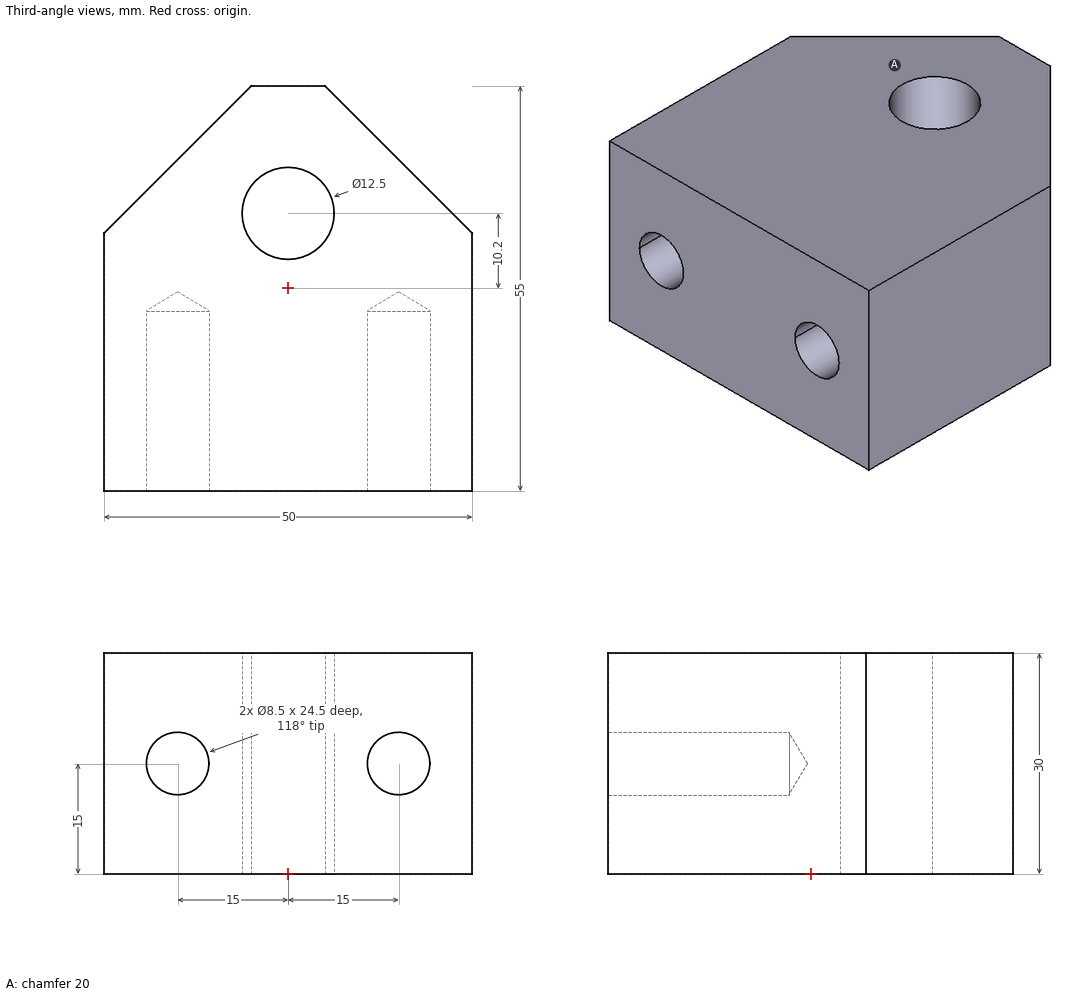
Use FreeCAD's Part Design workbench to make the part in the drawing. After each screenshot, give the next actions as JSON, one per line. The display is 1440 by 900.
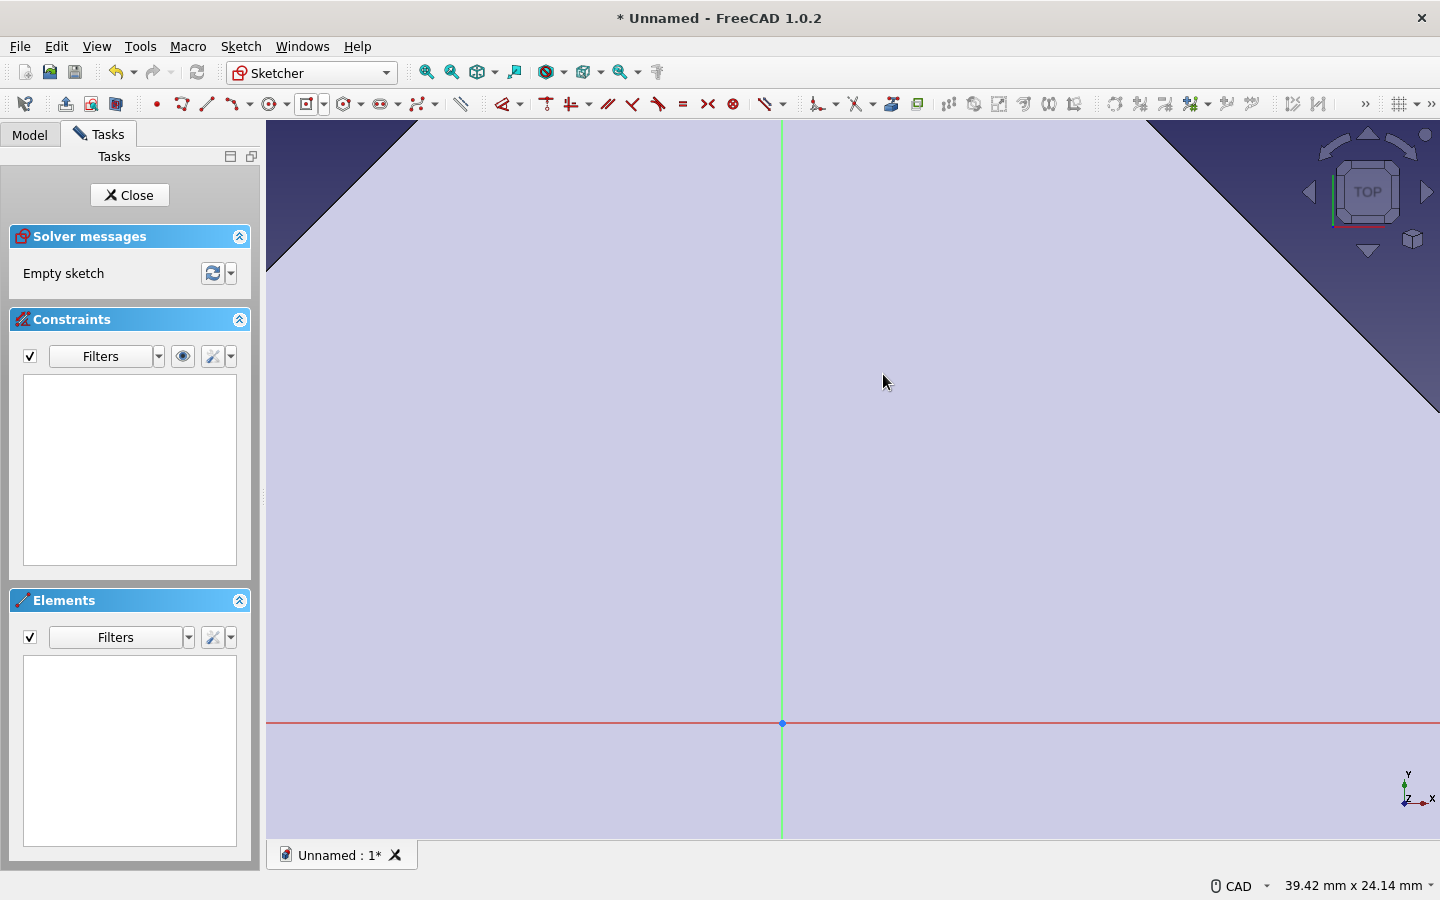
{"action": "left_click", "coordinate": [268, 104]}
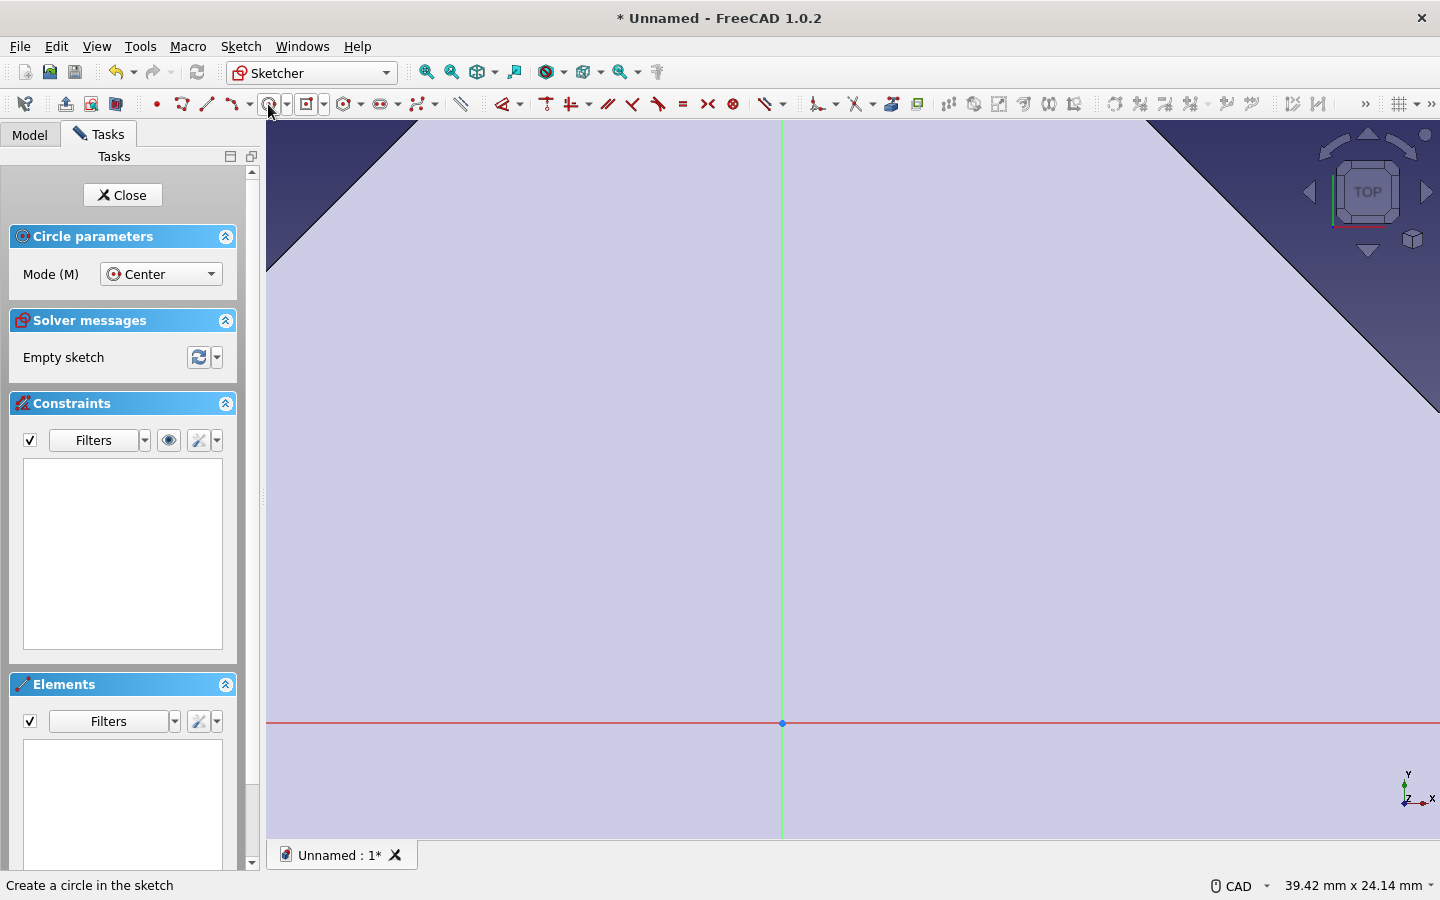
{"action": "left_click", "coordinate": [782, 420]}
{"action": "mouse_move", "coordinate": [914, 288]}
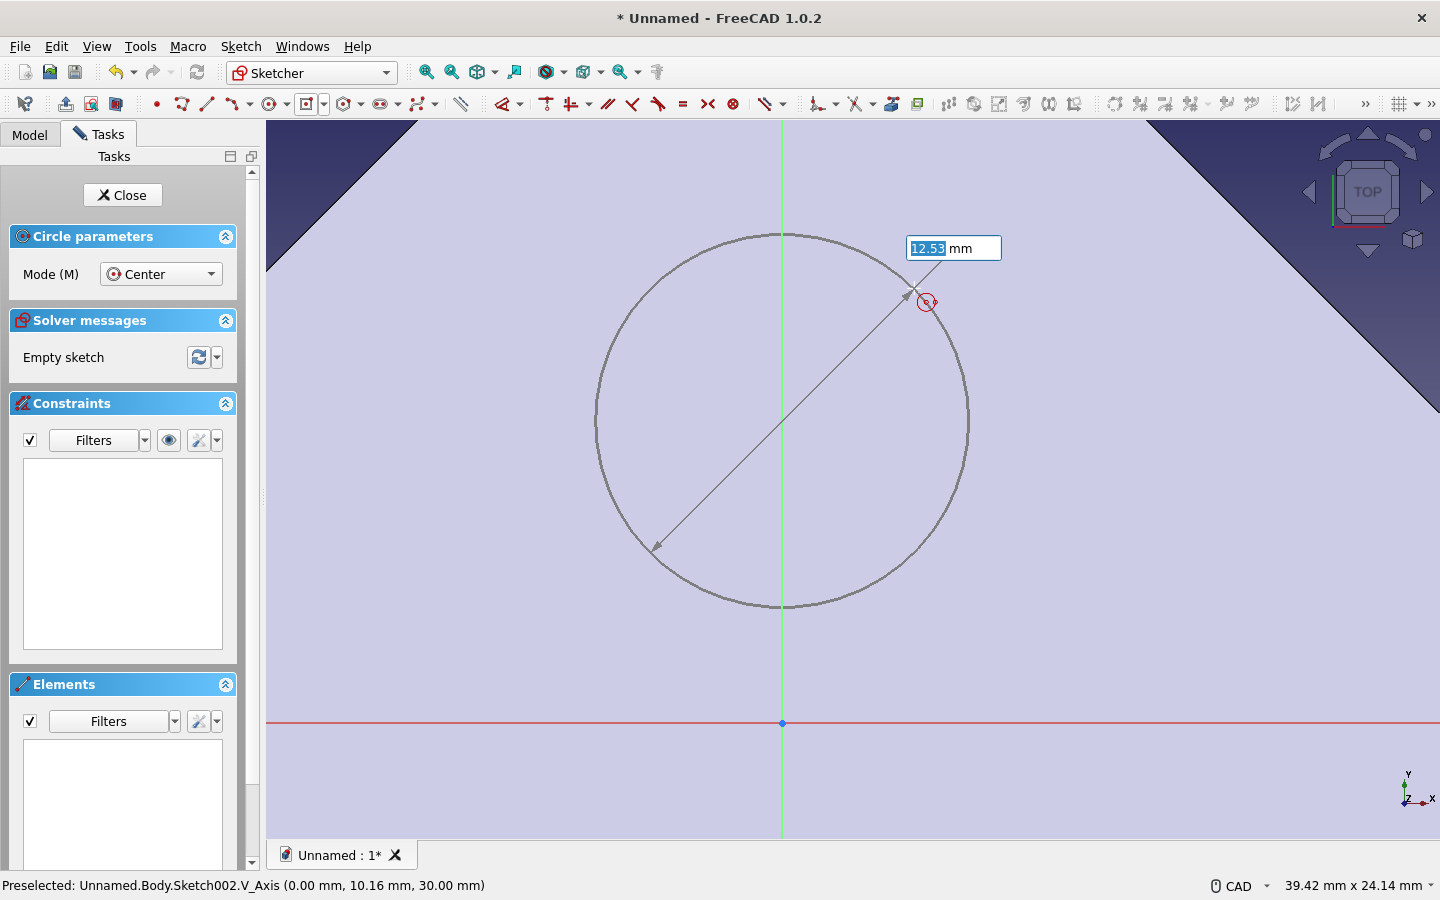
{"action": "type", "text": "12.5"}
{"action": "key", "text": "Return"}
{"action": "key", "text": "Escape"}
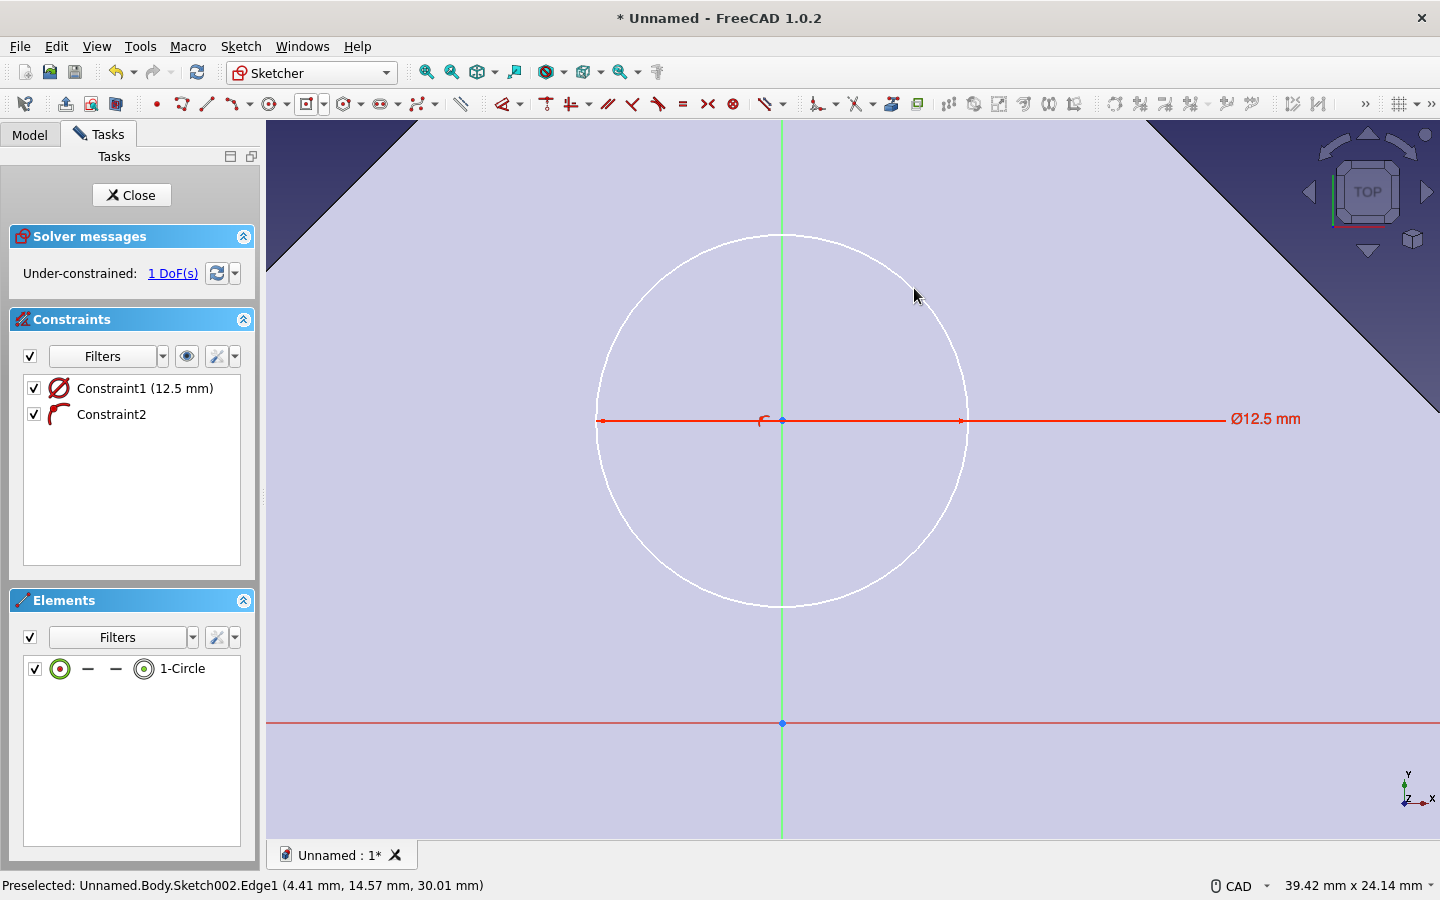
{"action": "left_click", "coordinate": [502, 104]}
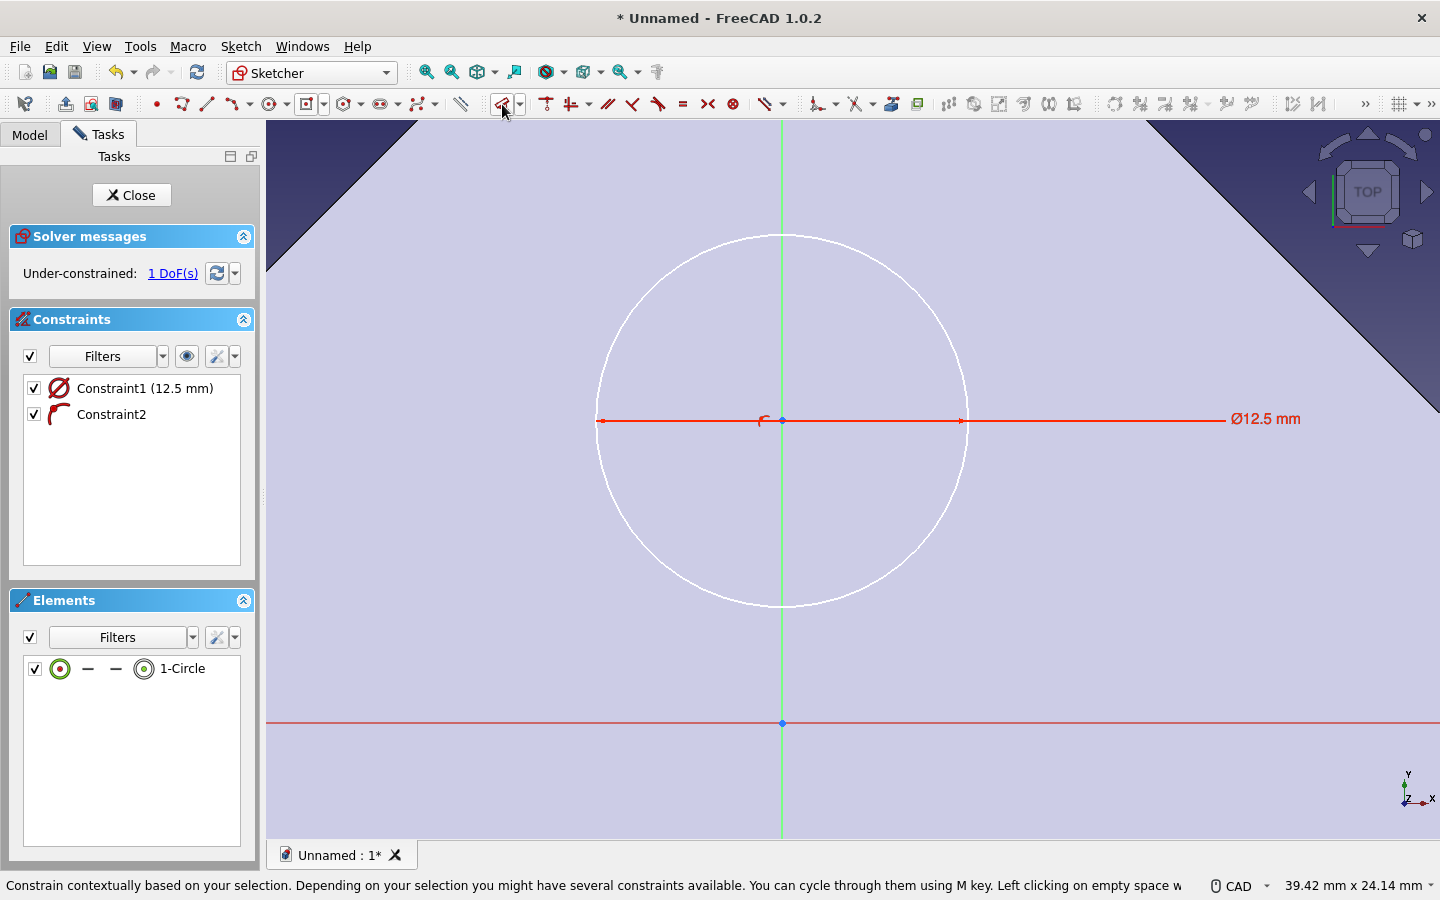
{"action": "left_click", "coordinate": [782, 421]}
{"action": "left_click", "coordinate": [816, 572]}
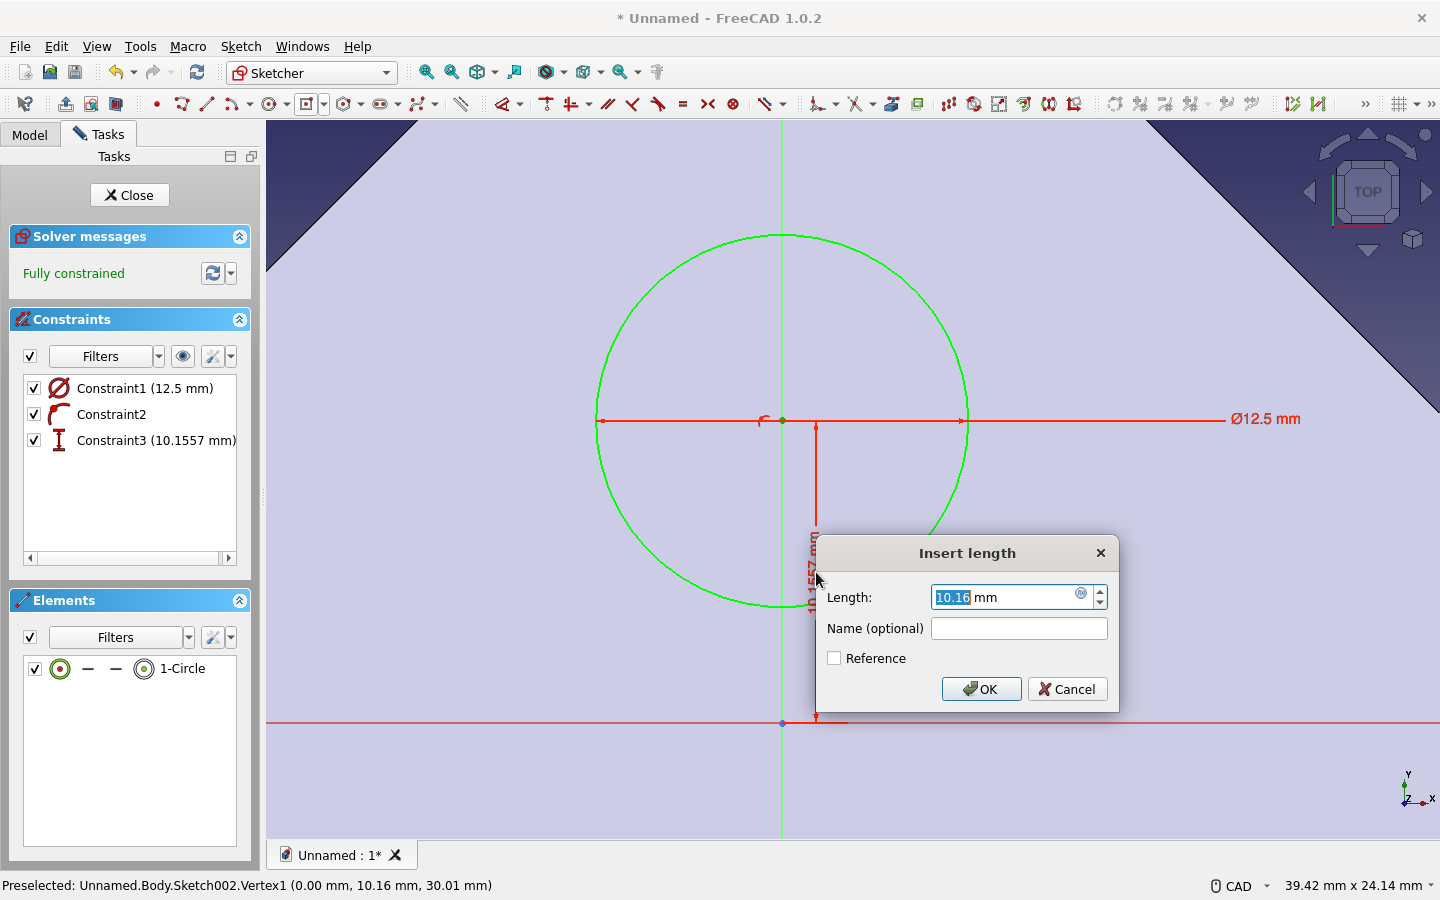
{"action": "type", "text": "10.2"}
{"action": "key", "text": "Return"}
{"action": "key", "text": "Escape"}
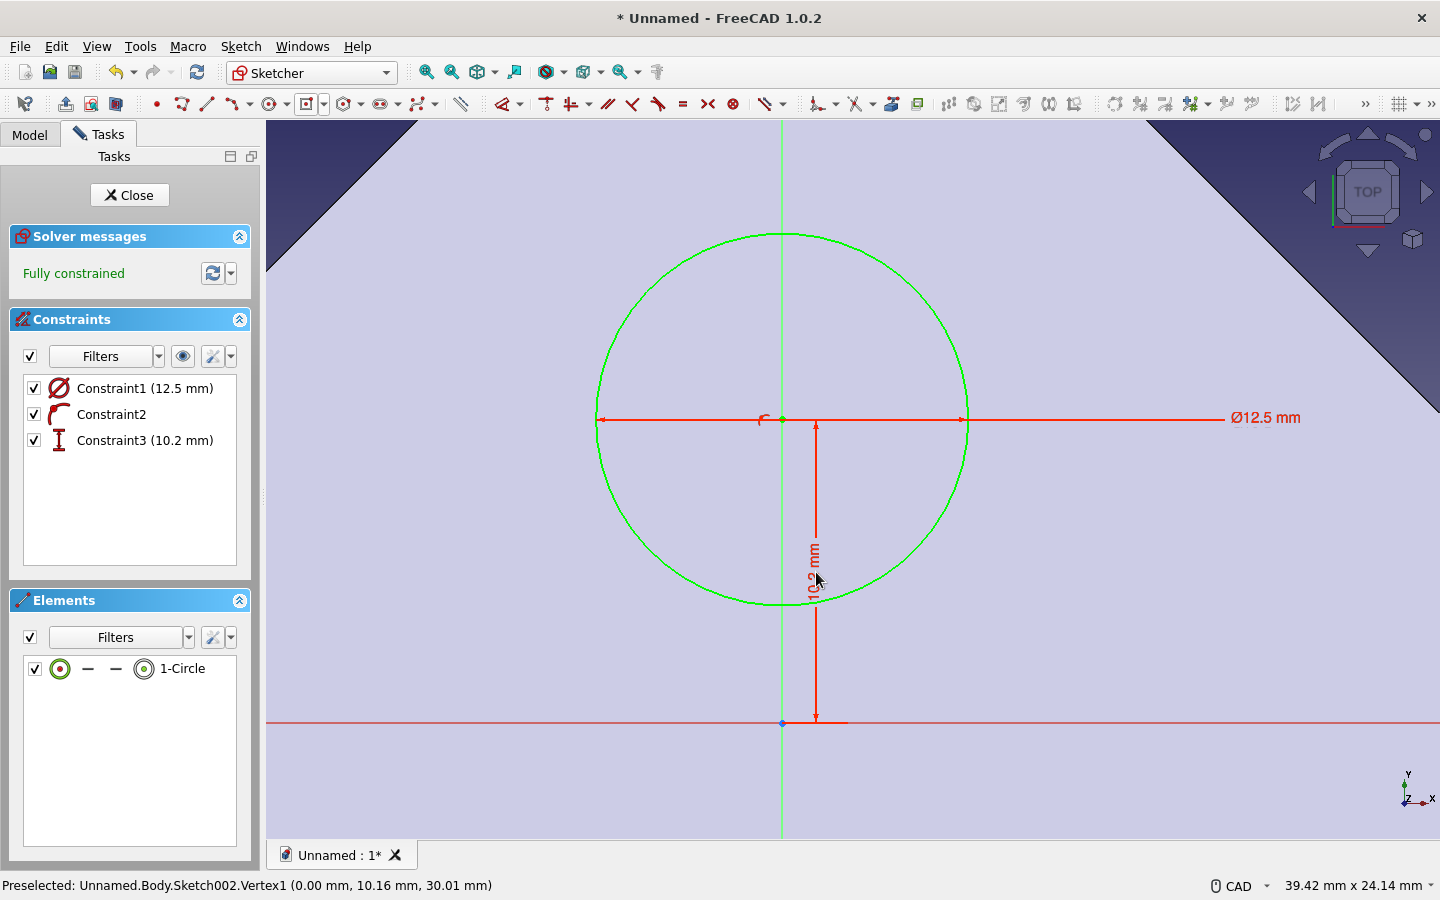
{"action": "left_click", "coordinate": [130, 195]}